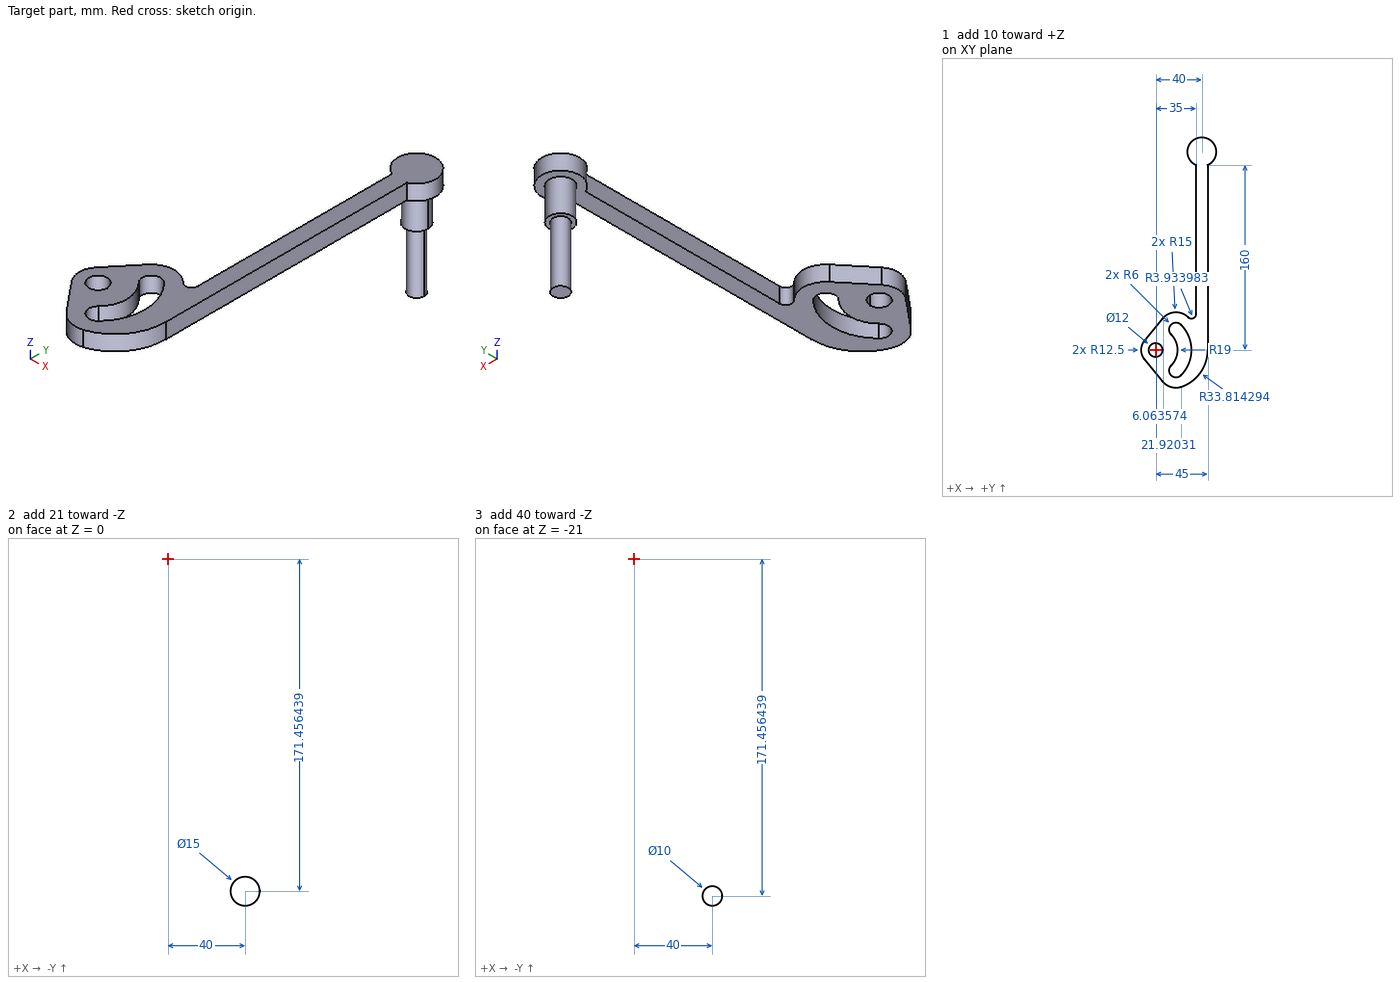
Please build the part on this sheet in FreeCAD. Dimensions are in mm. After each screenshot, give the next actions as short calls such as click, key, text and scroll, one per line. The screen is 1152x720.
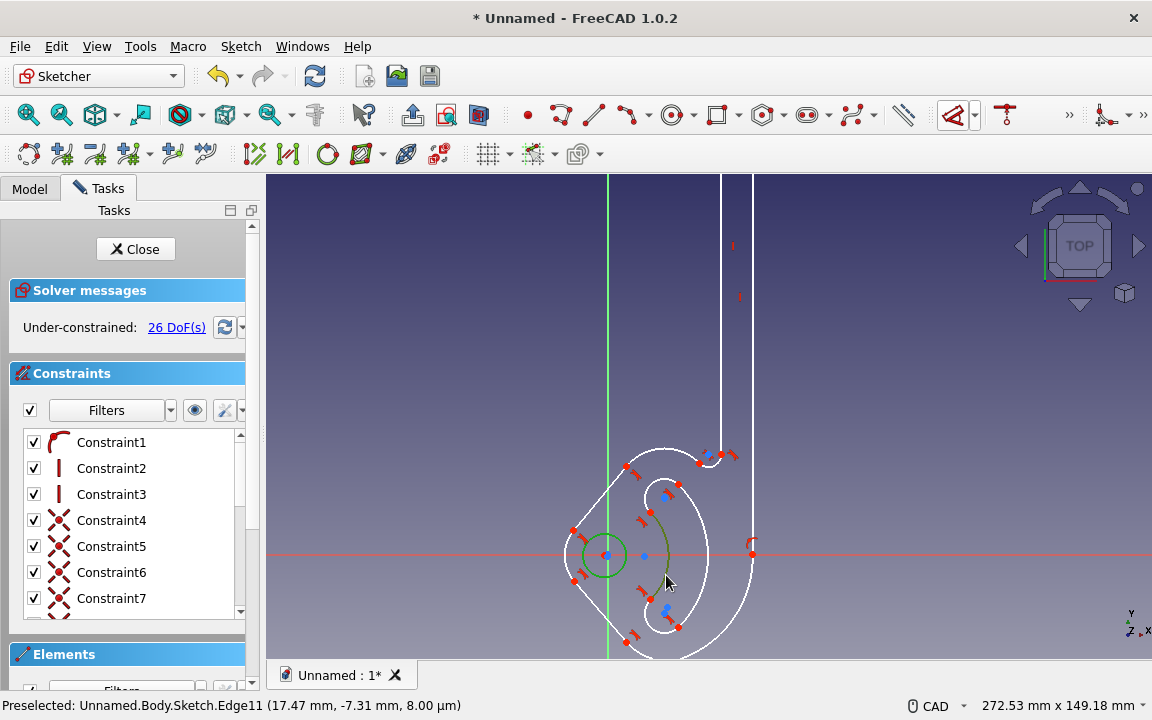
click(1005, 116)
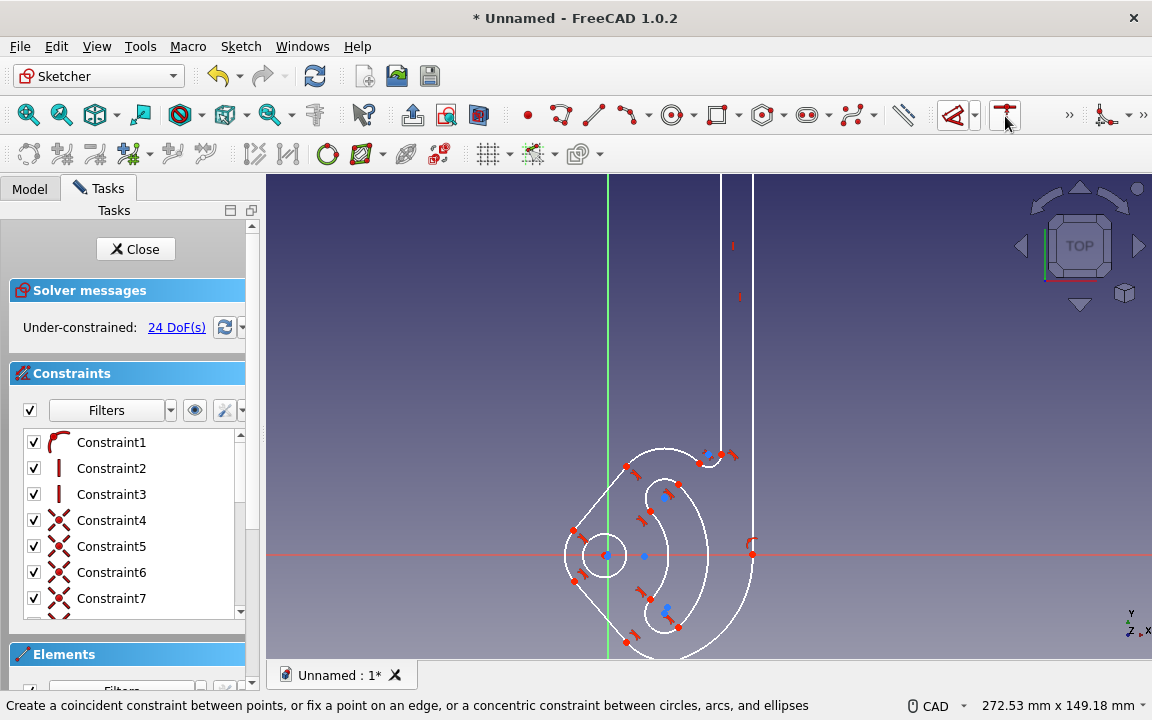
click(679, 451)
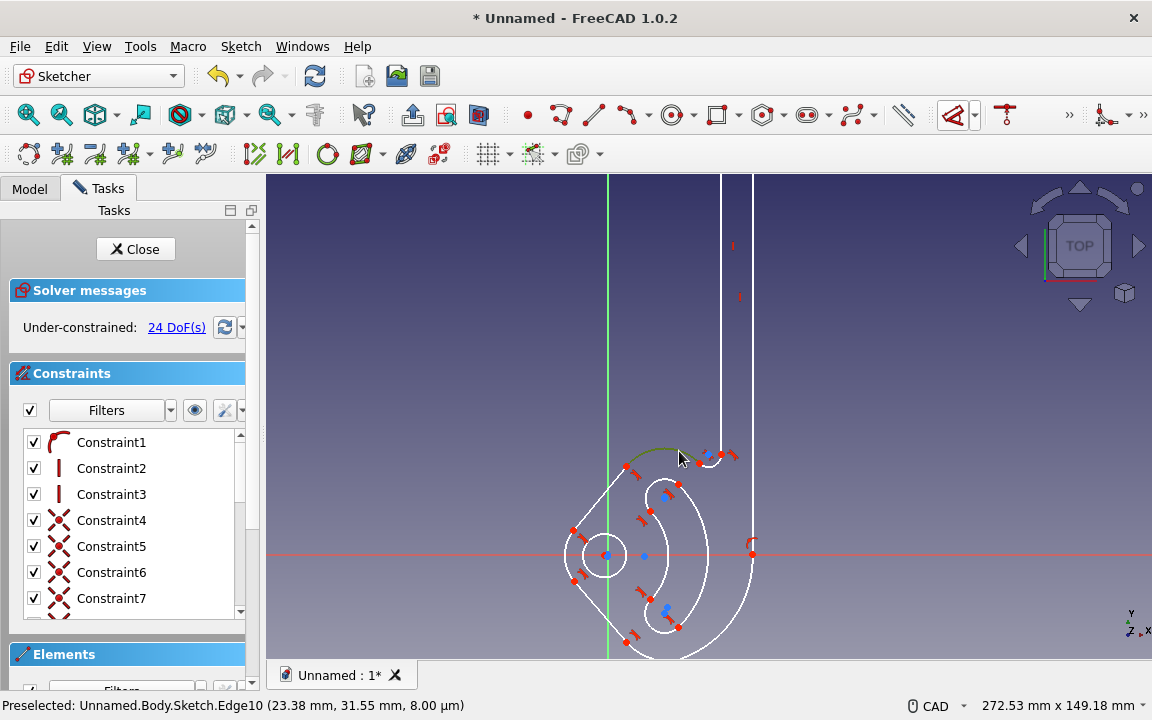
click(662, 479)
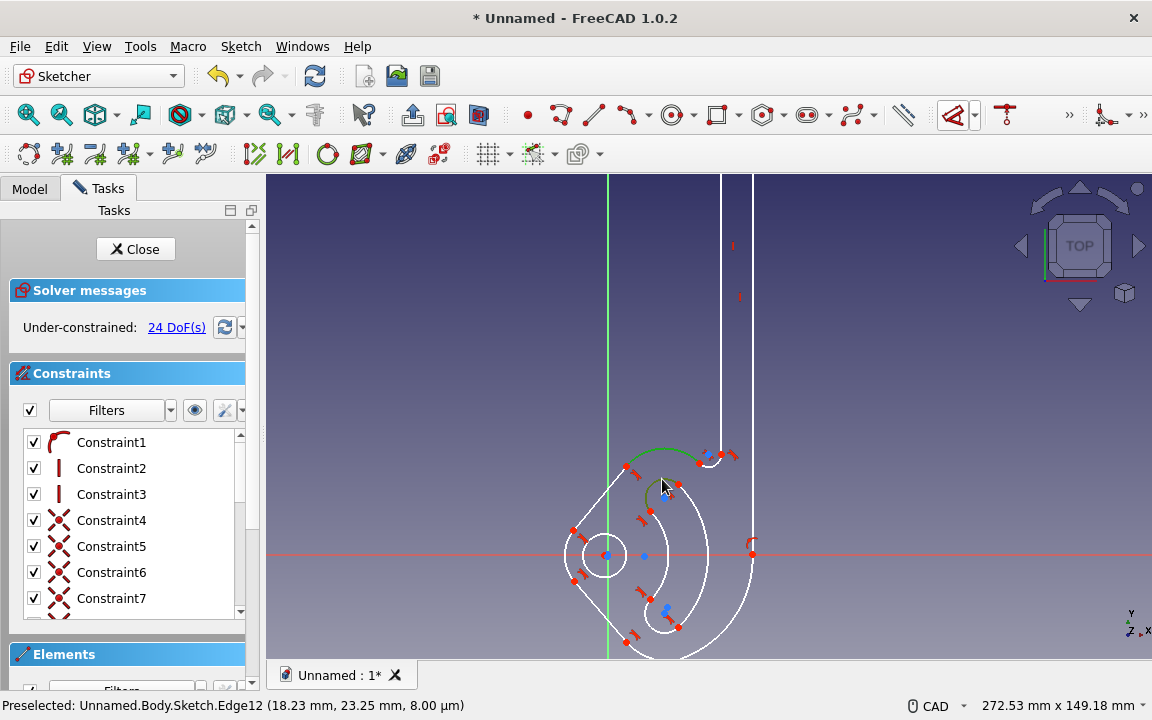
click(1005, 116)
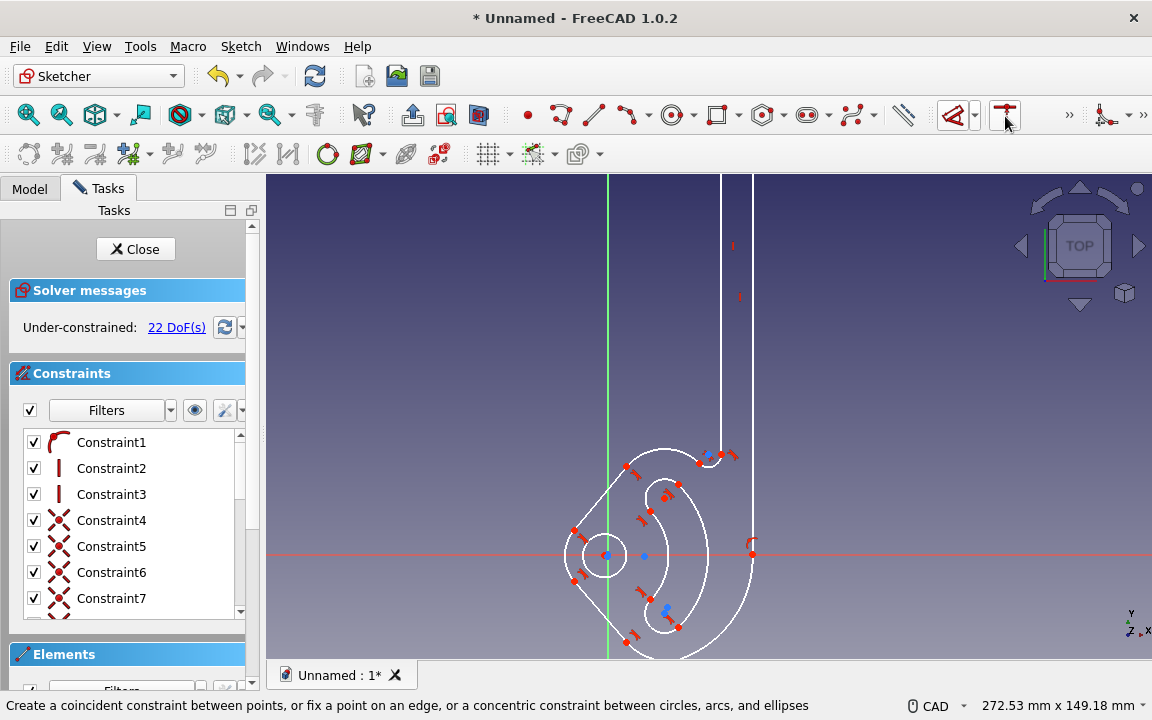
click(620, 540)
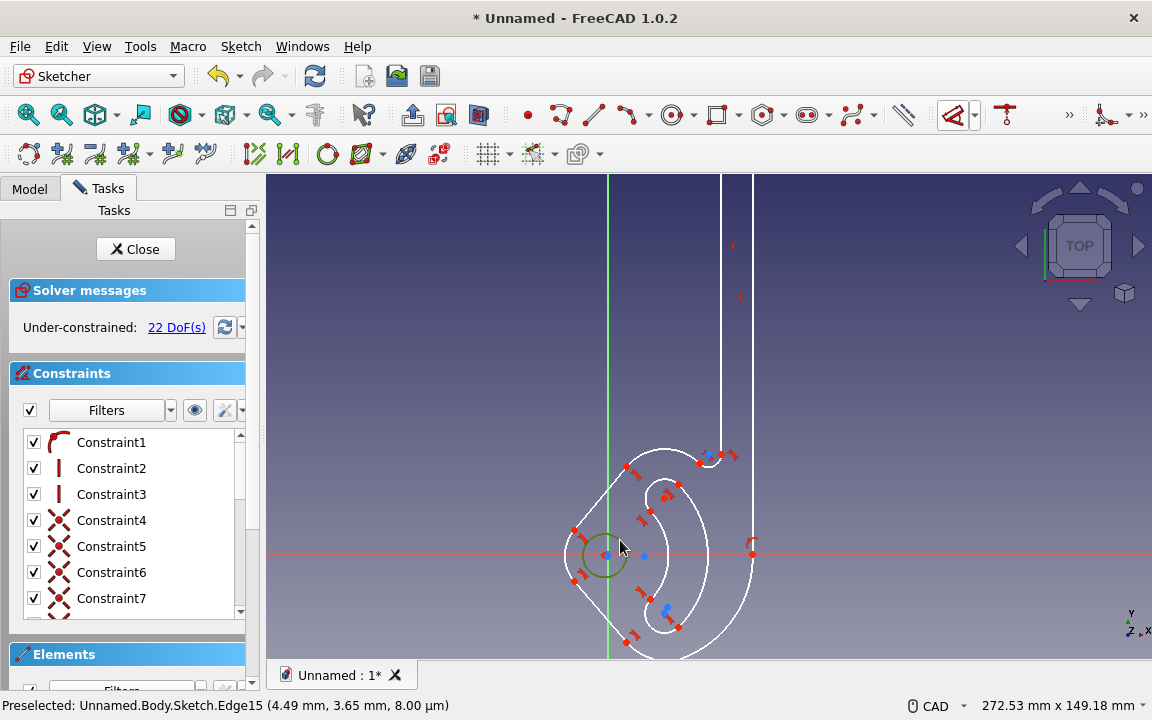
click(703, 587)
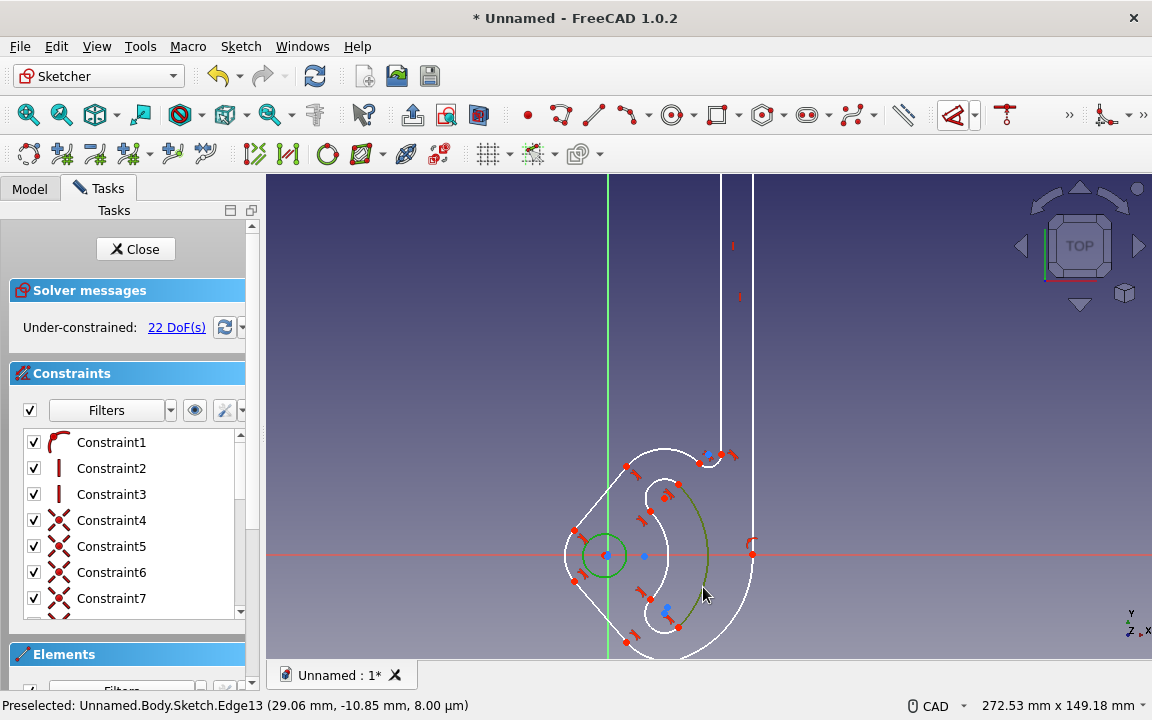
key(c)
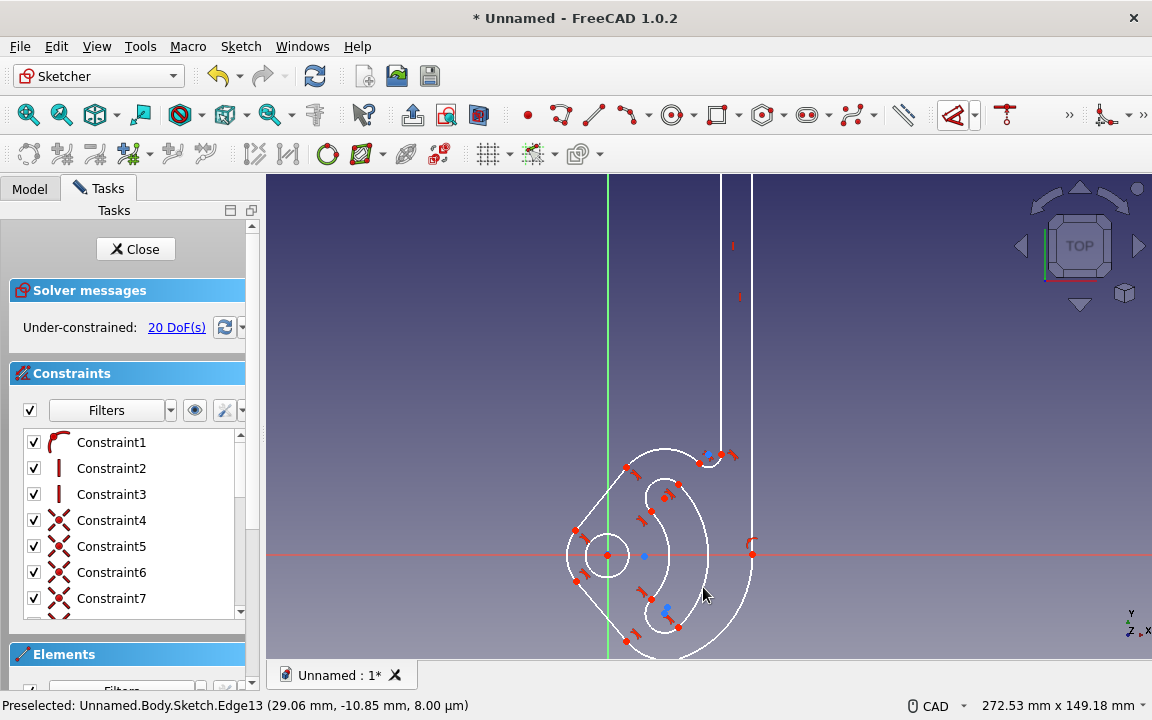
scroll(624, 505, down, 4)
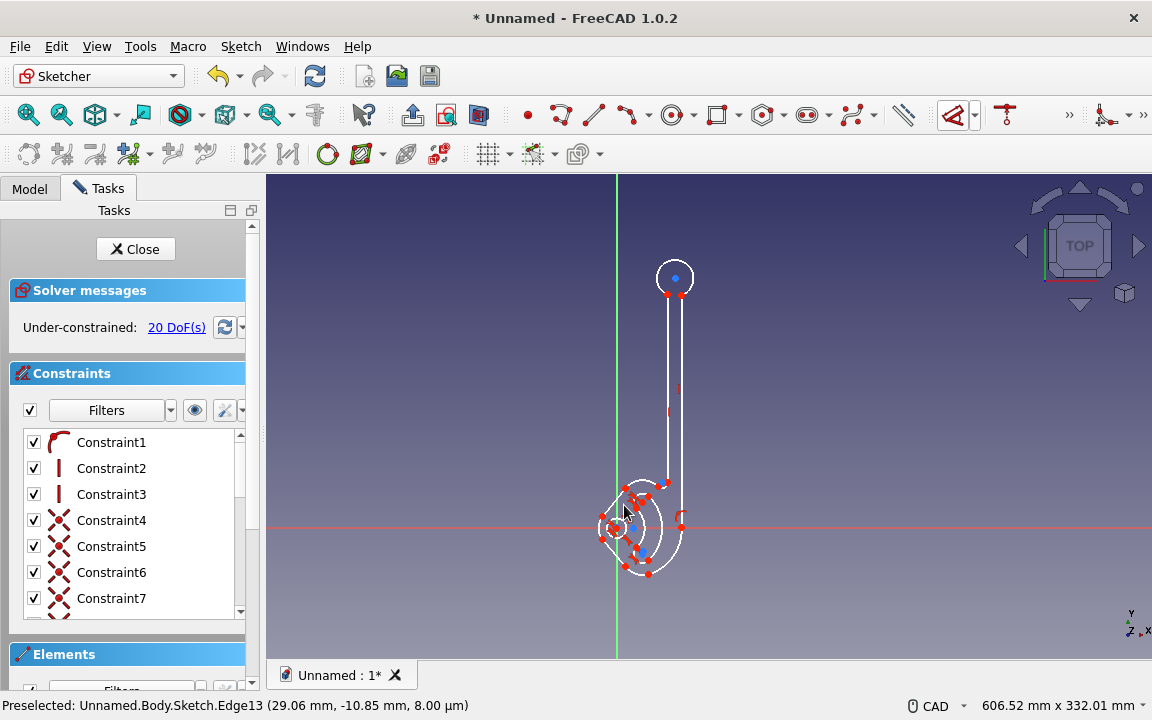
scroll(631, 572, up, 3)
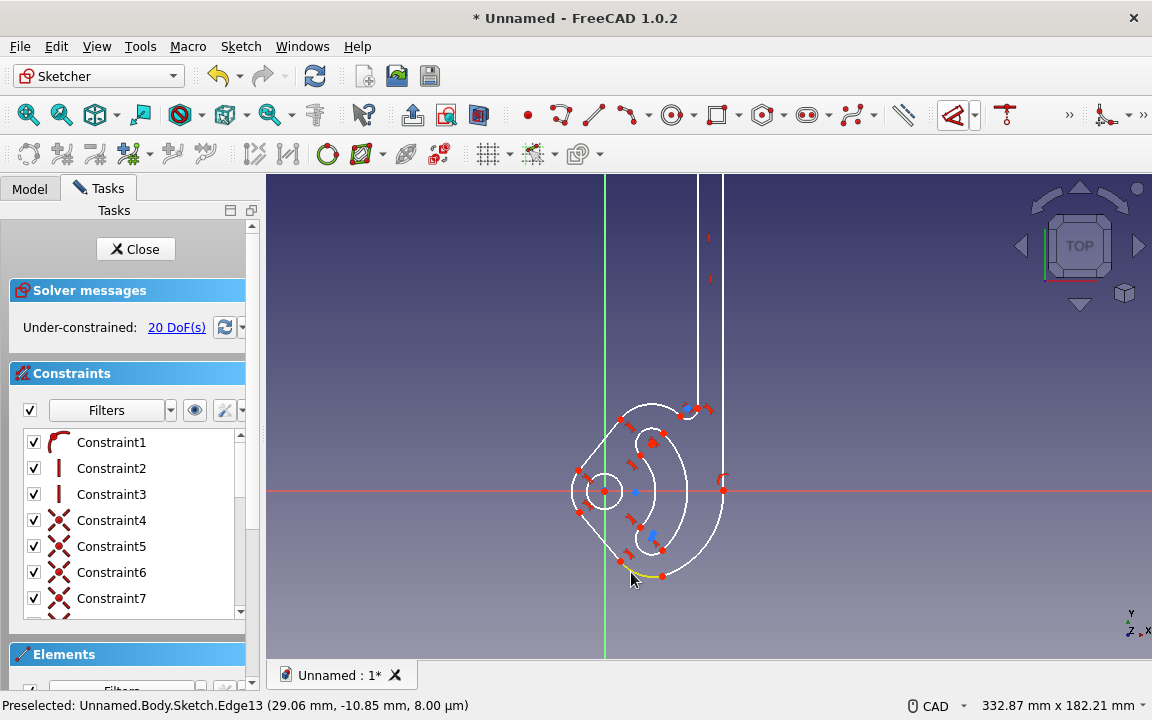
click(631, 571)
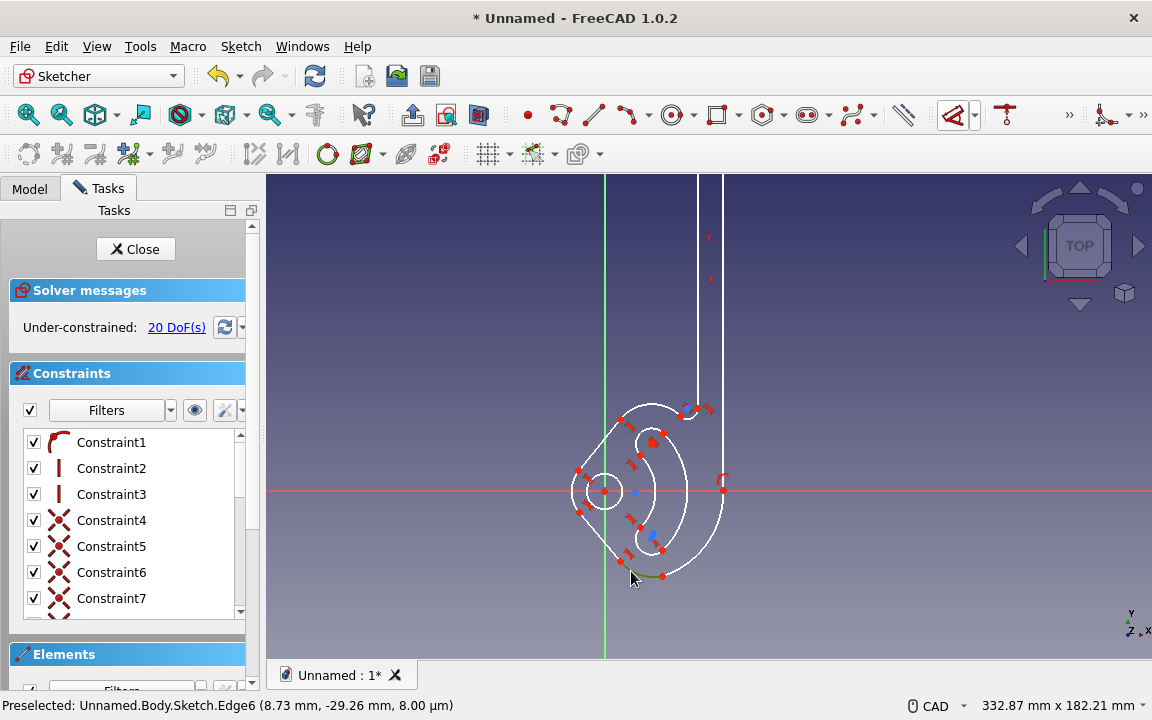
click(636, 541)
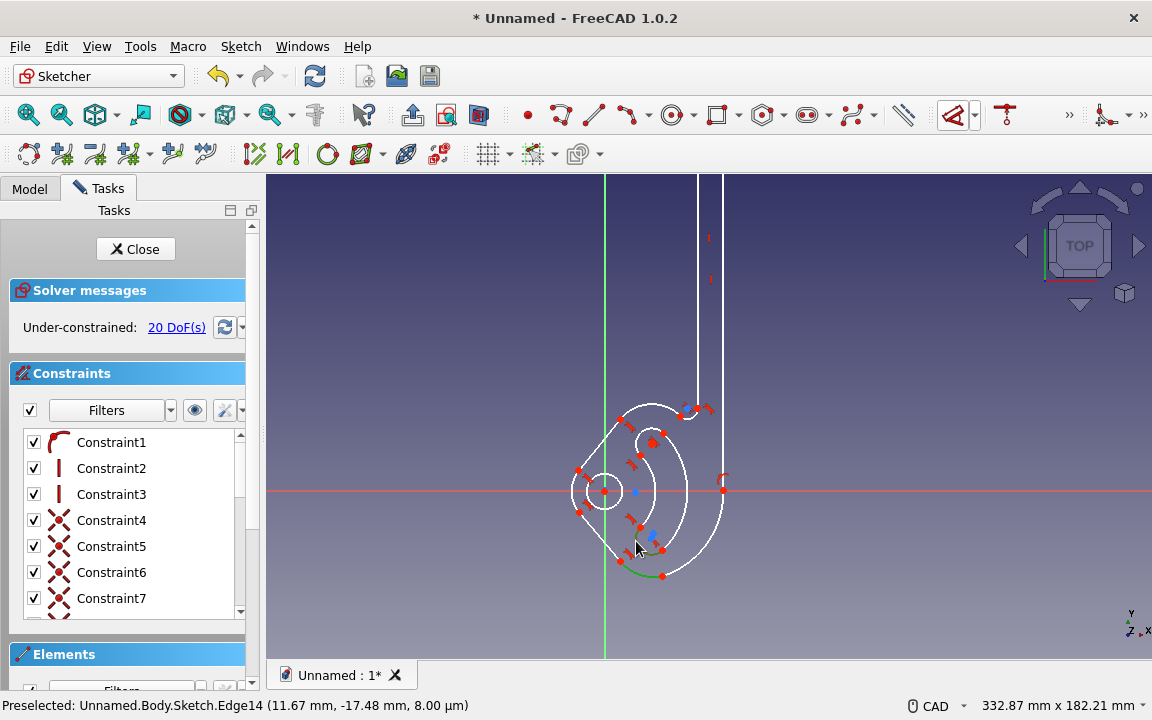
key(c)